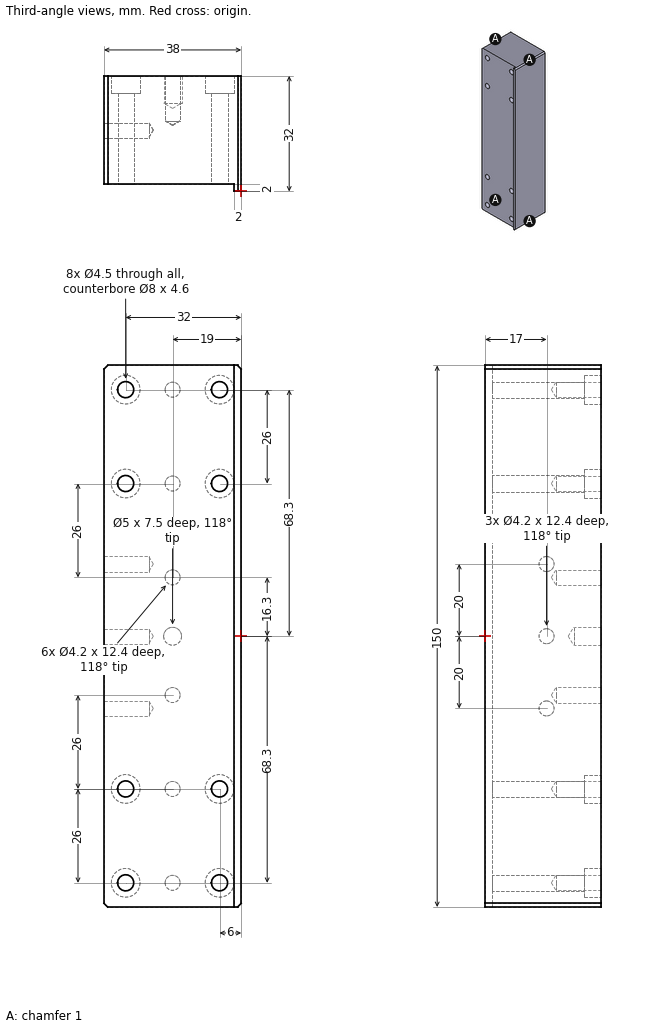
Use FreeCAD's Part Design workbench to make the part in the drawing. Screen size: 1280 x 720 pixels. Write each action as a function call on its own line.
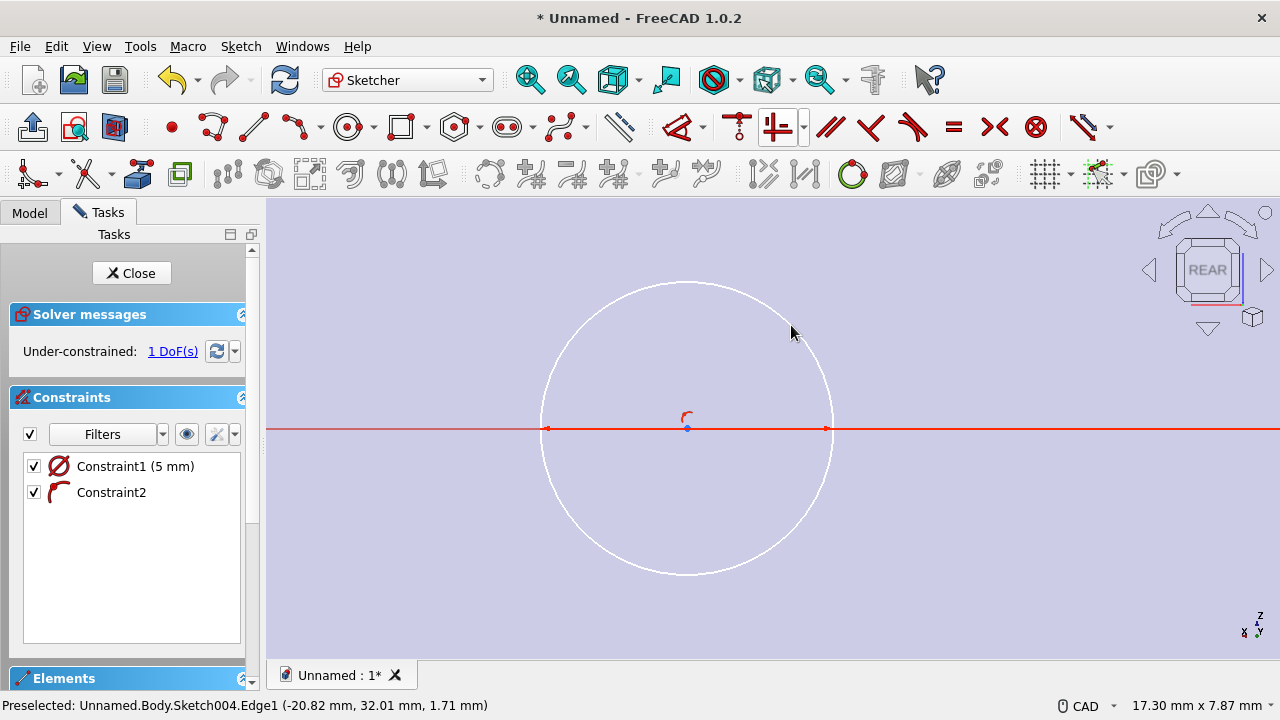
click(676, 128)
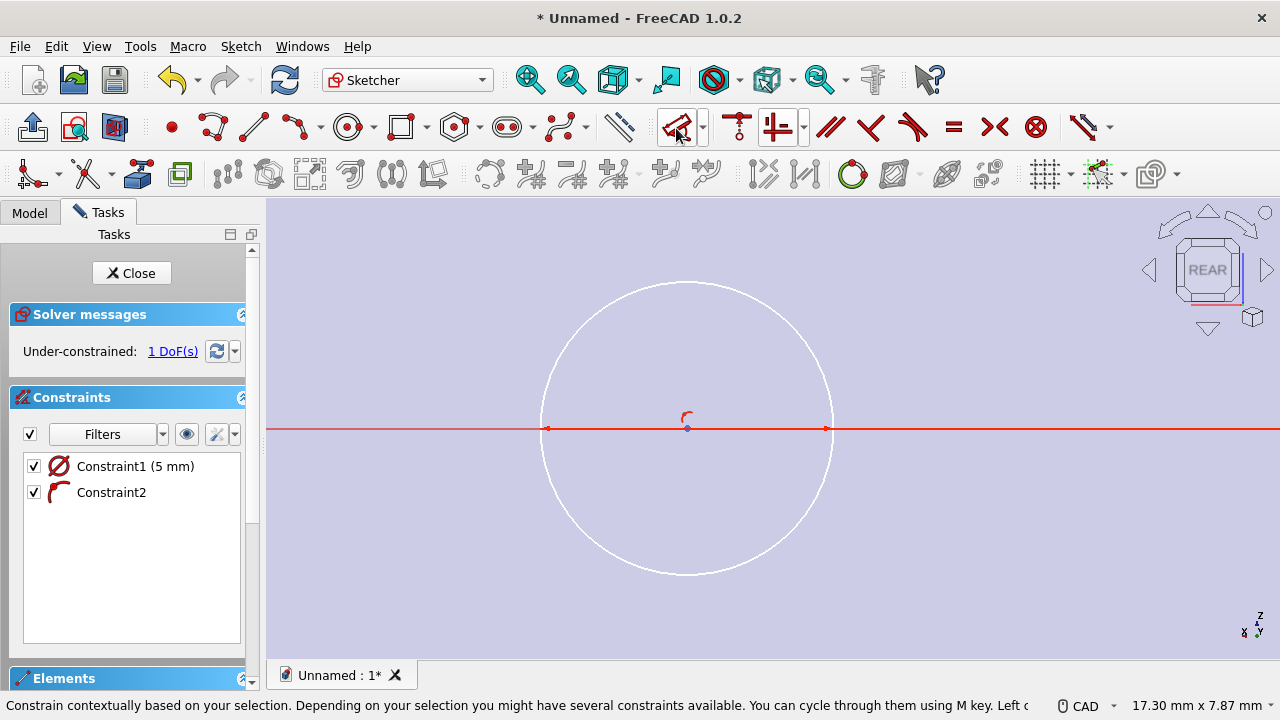
click(687, 428)
click(491, 462)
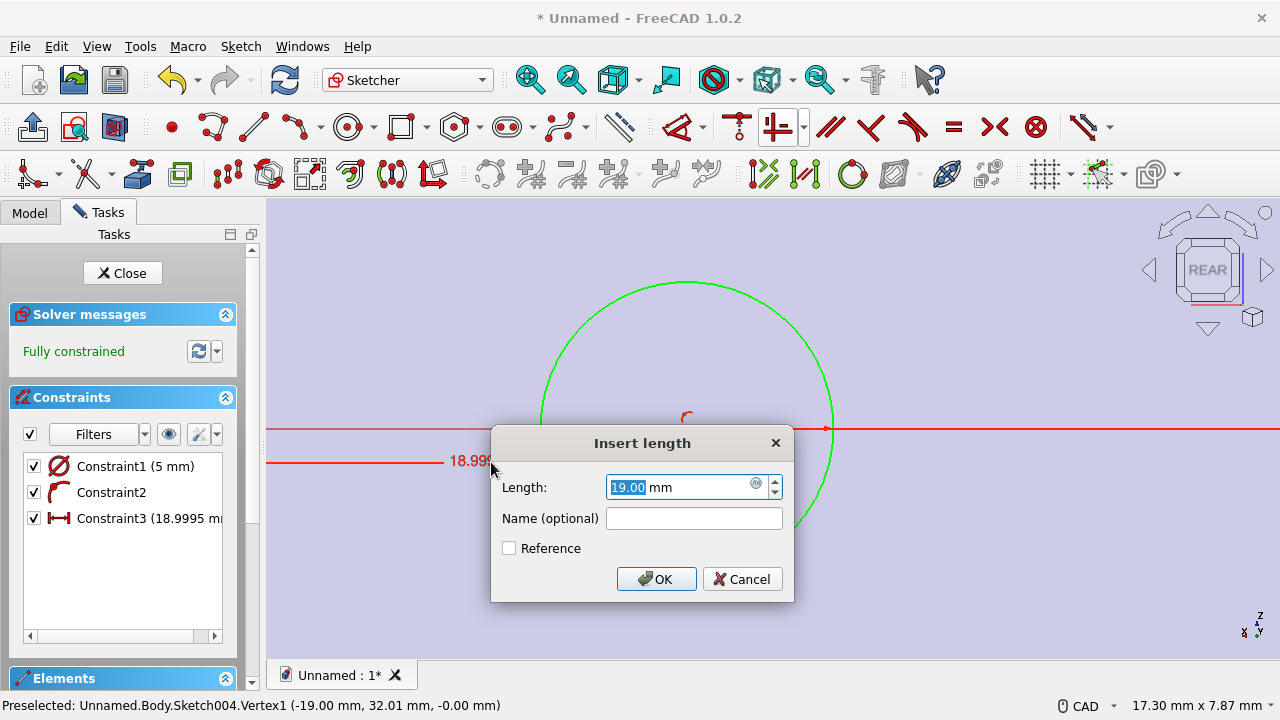
text(19)
key(Return)
key(Escape)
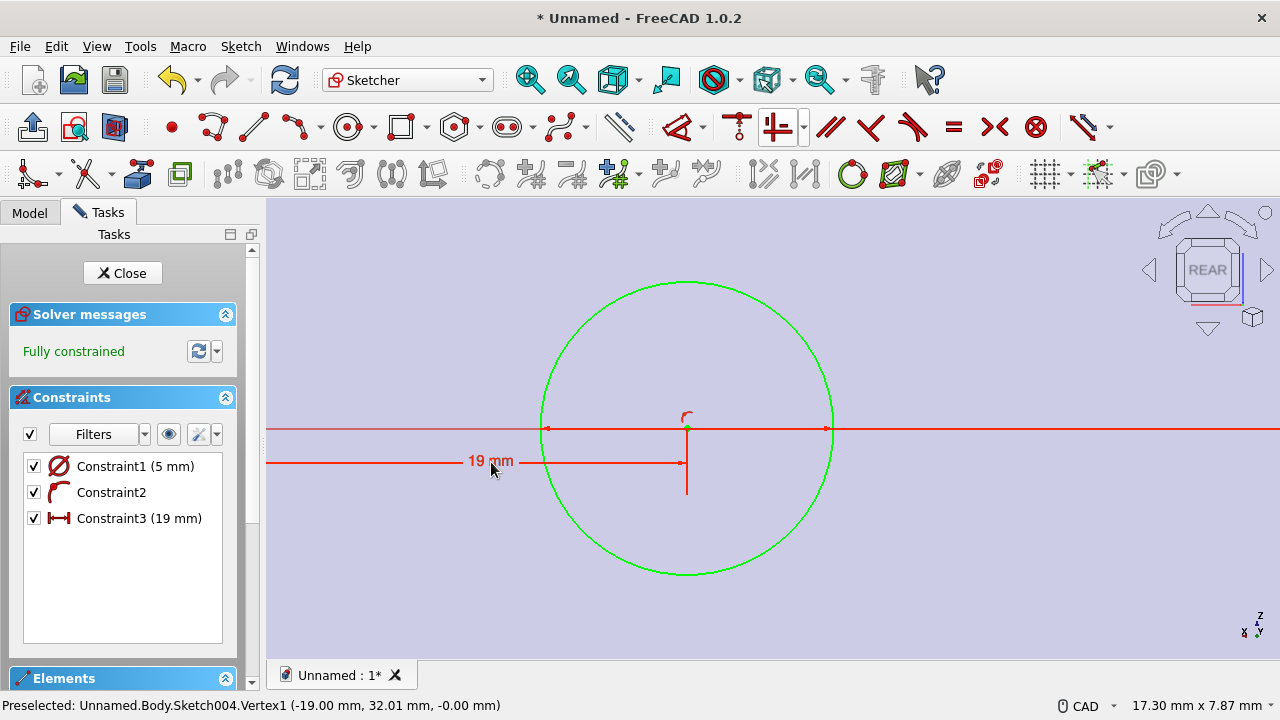
click(123, 273)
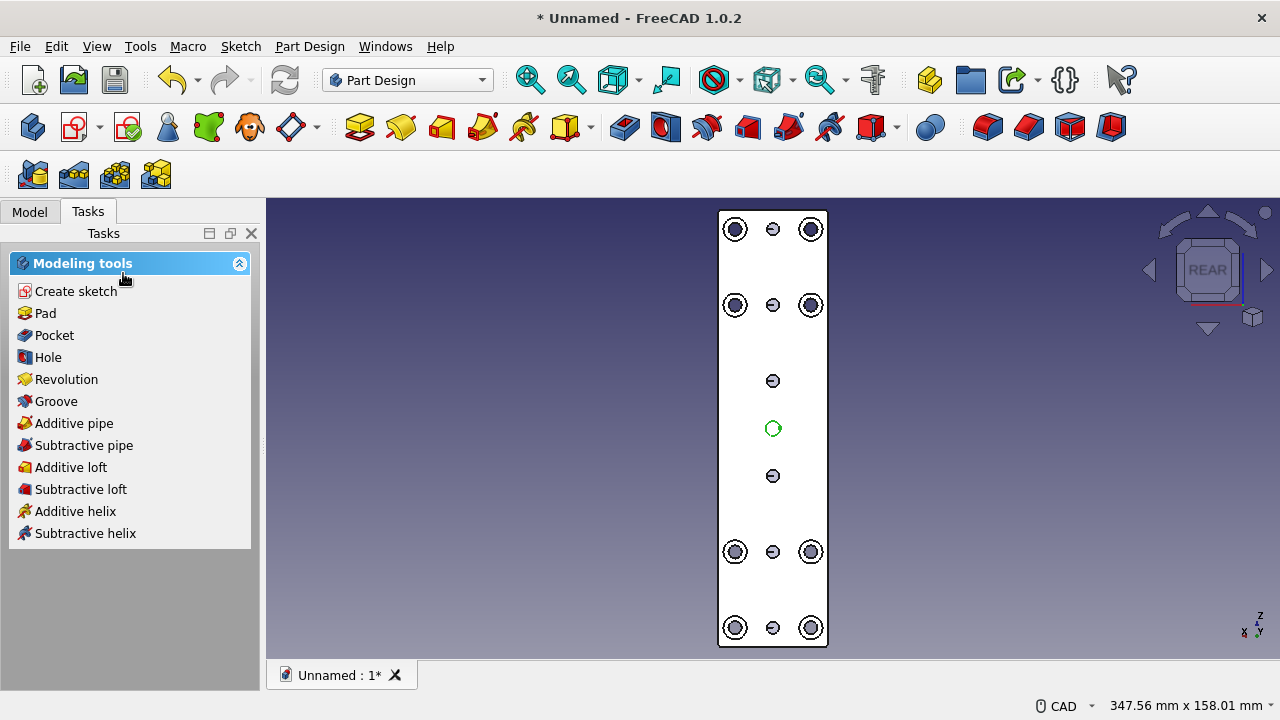
click(666, 128)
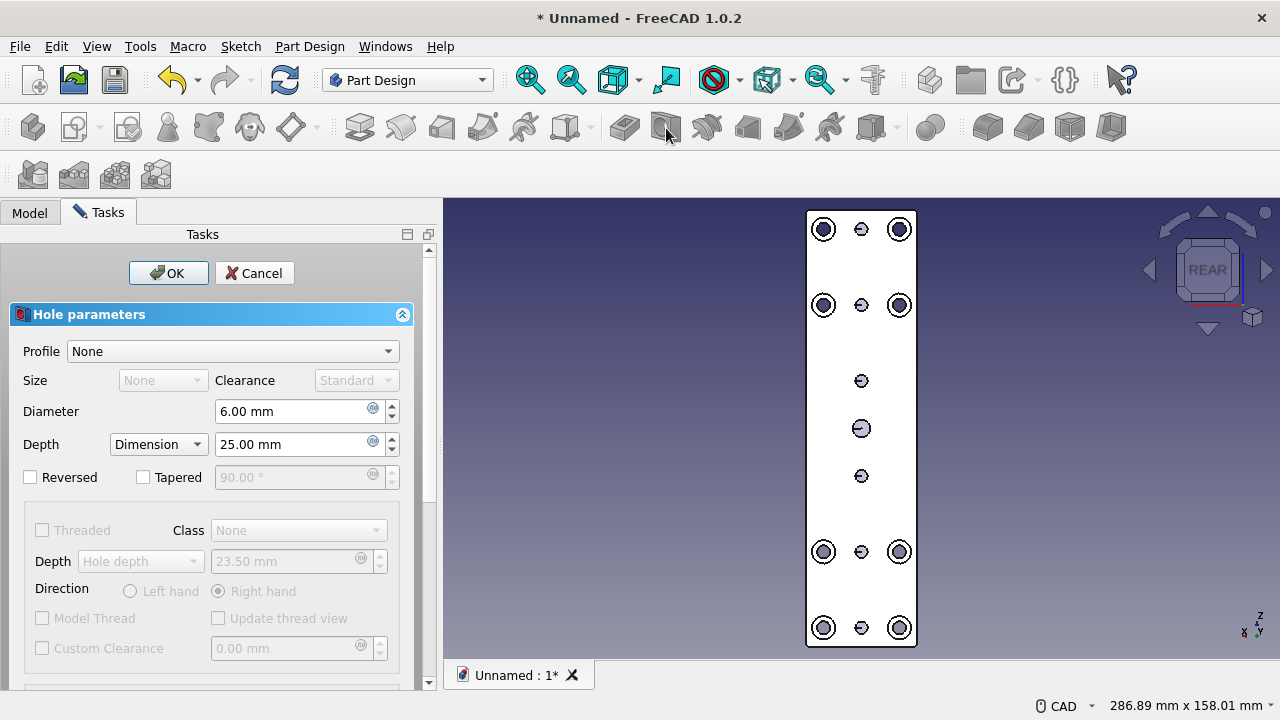
triple_click(300, 412)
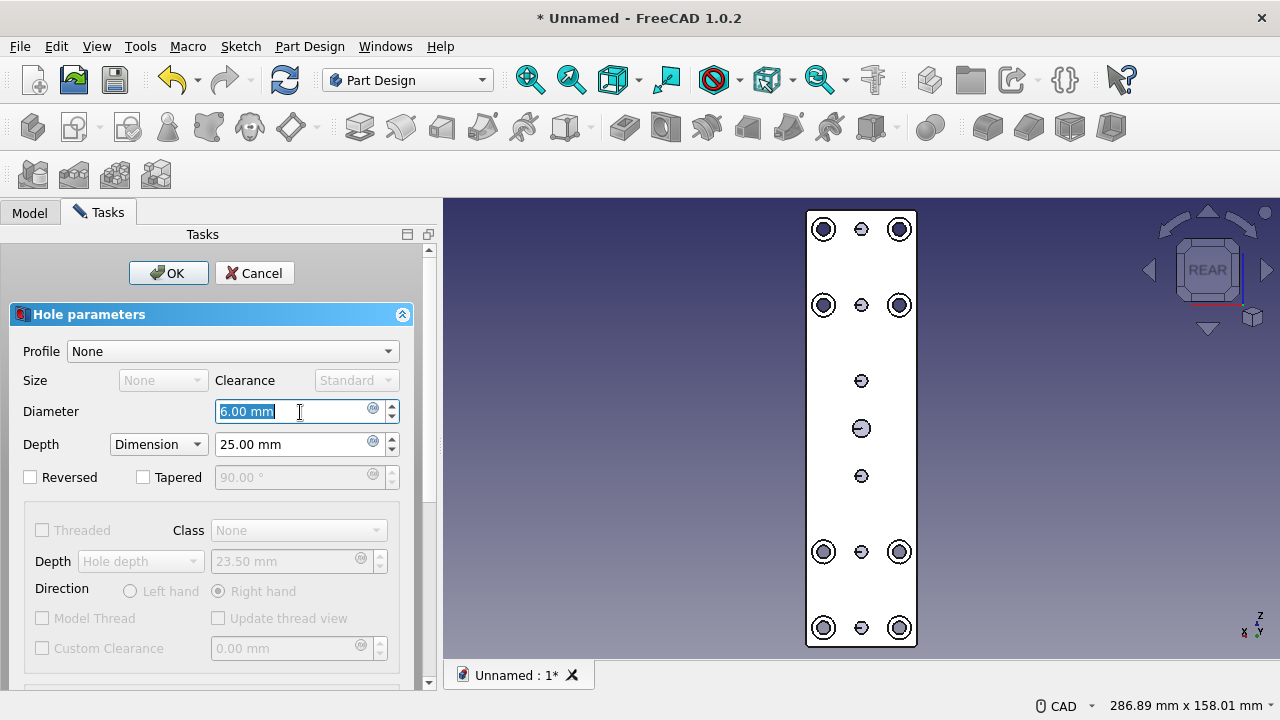
text(5)
key(Tab)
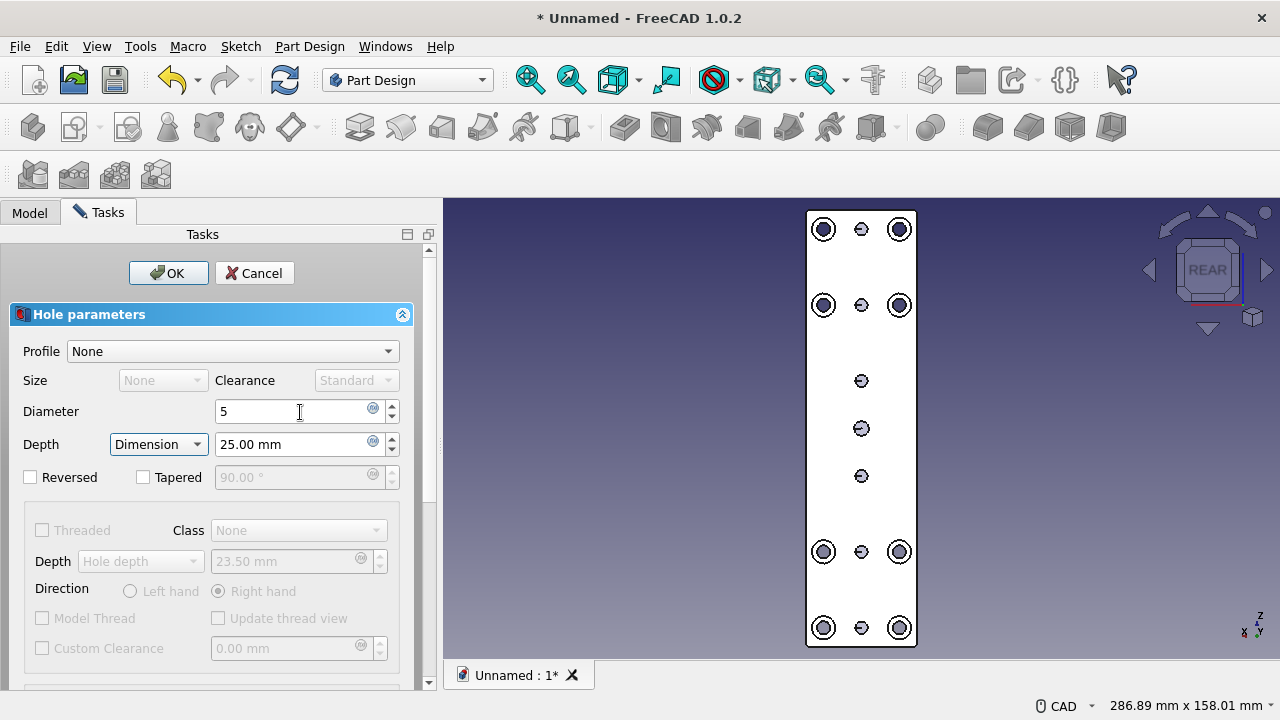
triple_click(300, 444)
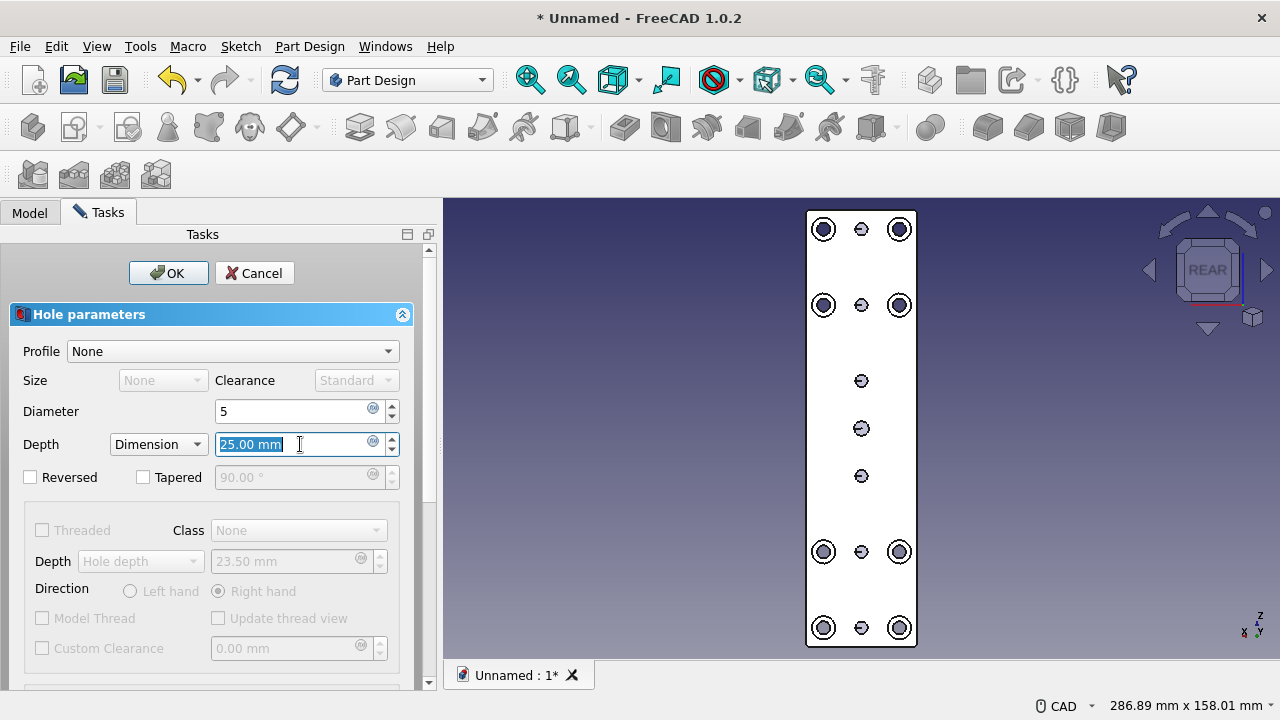
text(7.5)
key(Tab)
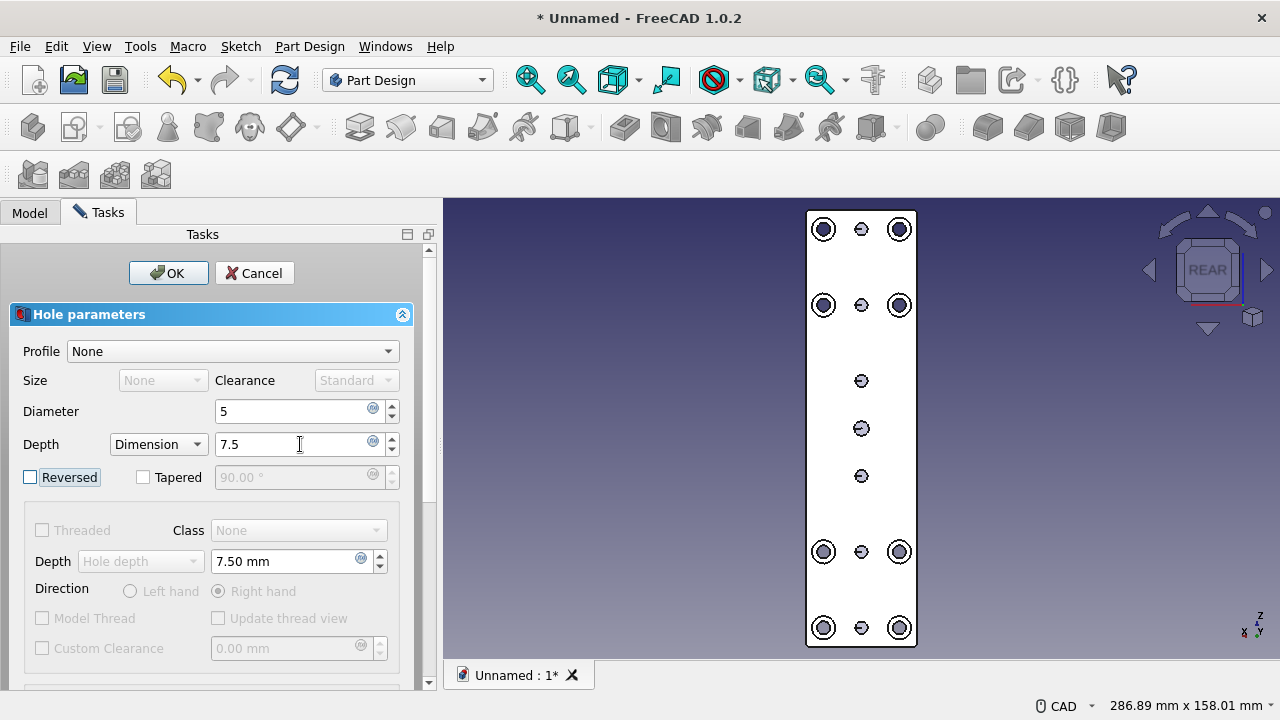
click(169, 273)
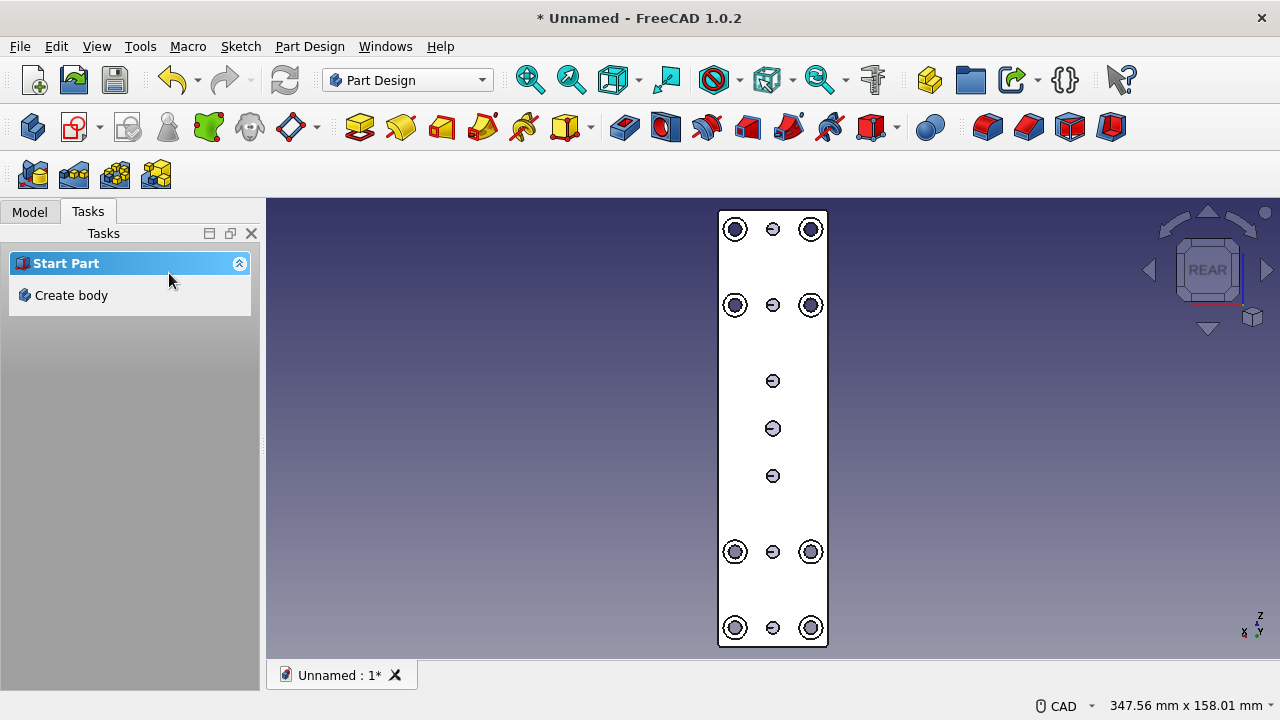
key(0)